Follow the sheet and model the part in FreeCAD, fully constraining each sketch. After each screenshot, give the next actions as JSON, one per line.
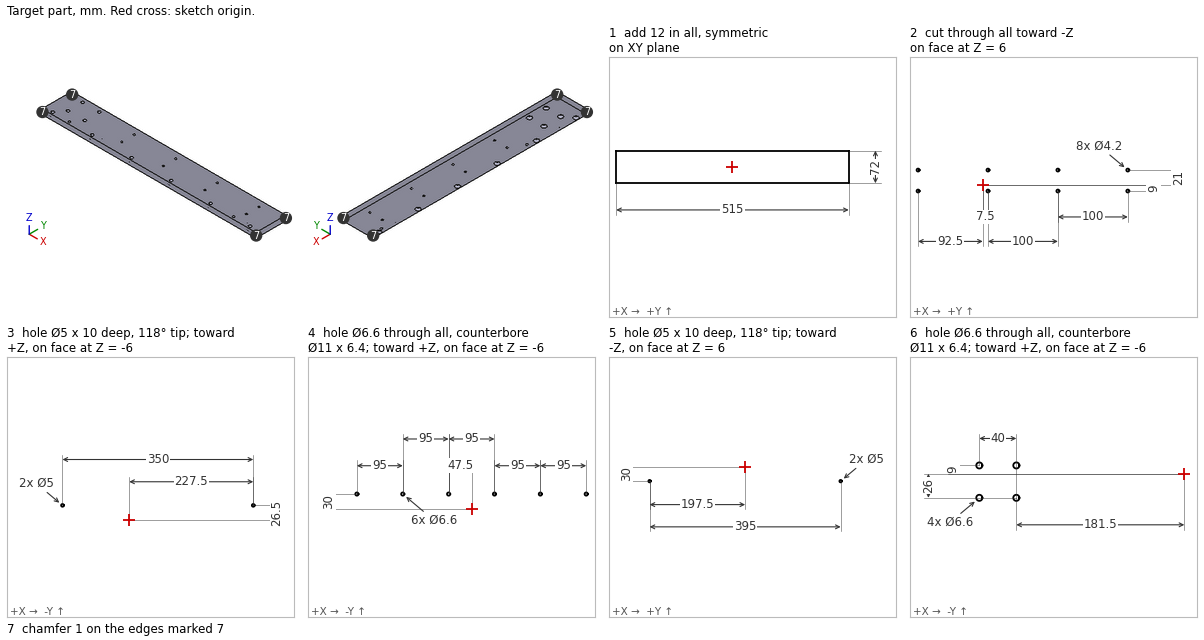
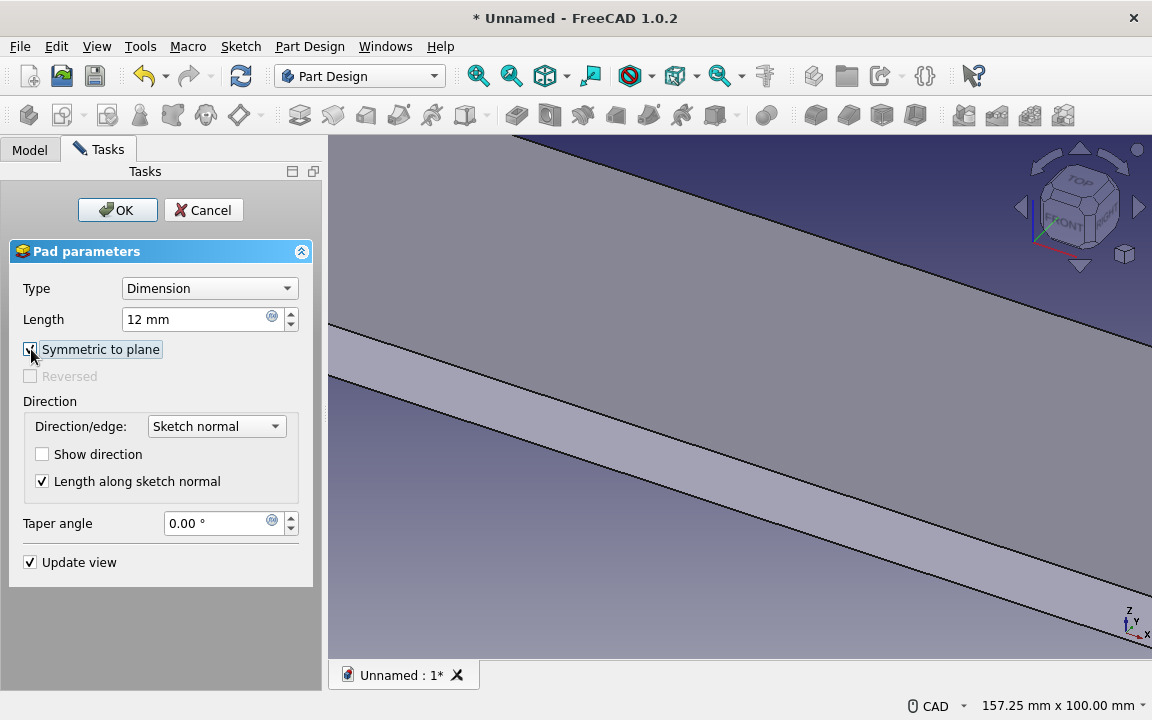
{"action": "left_click", "coordinate": [118, 210]}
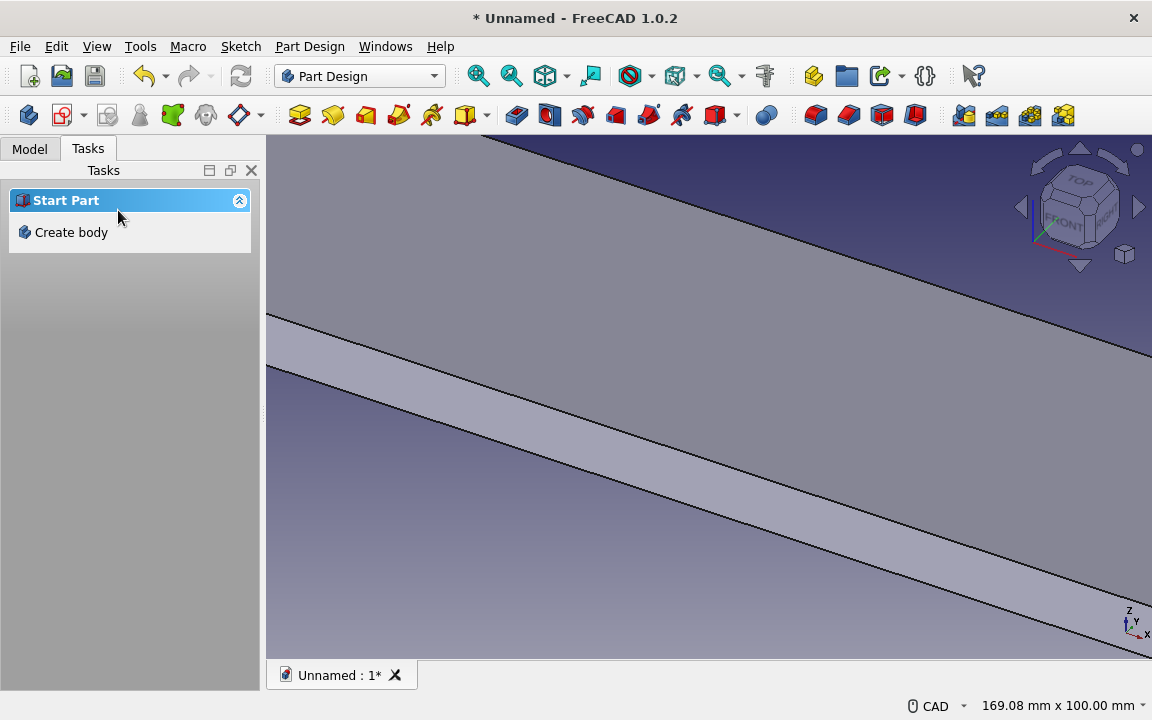
{"action": "left_click", "coordinate": [479, 76]}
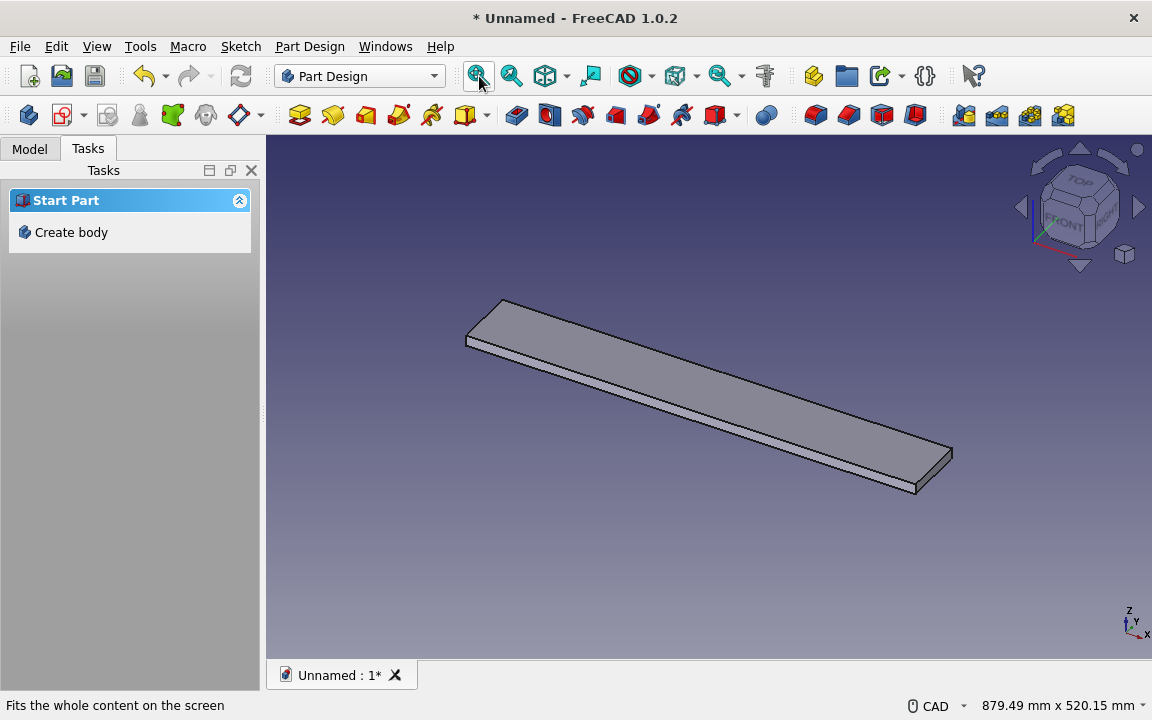
{"action": "left_click", "coordinate": [902, 455]}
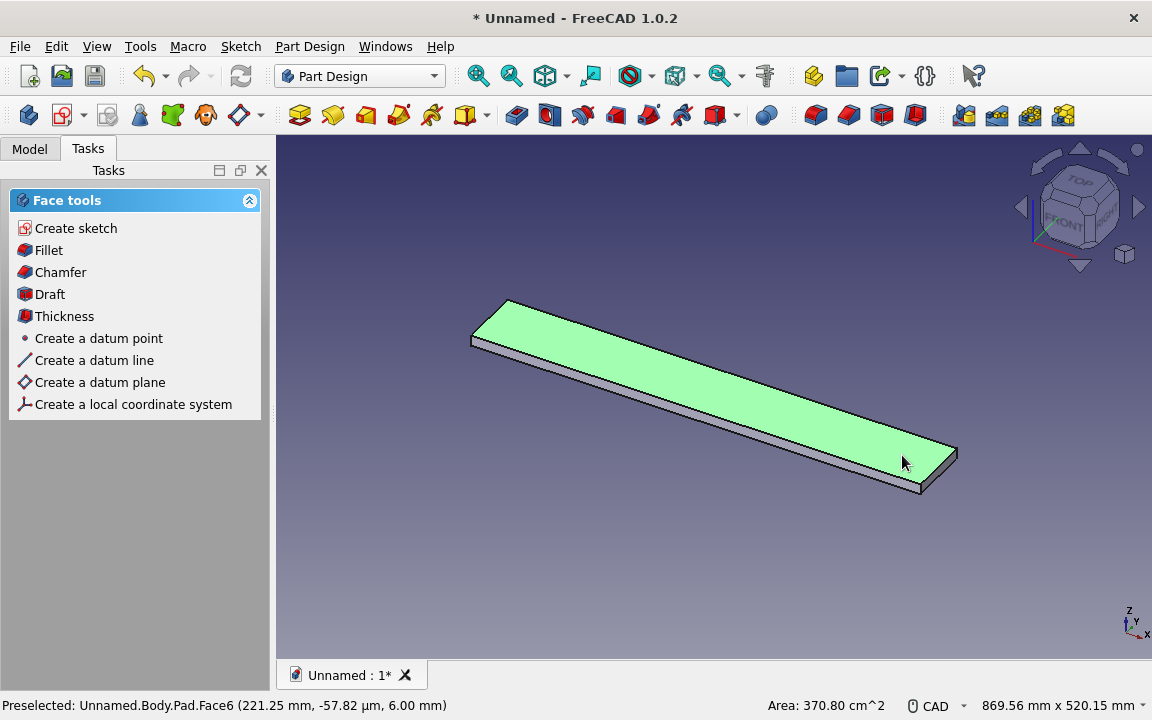
{"action": "left_click", "coordinate": [62, 116]}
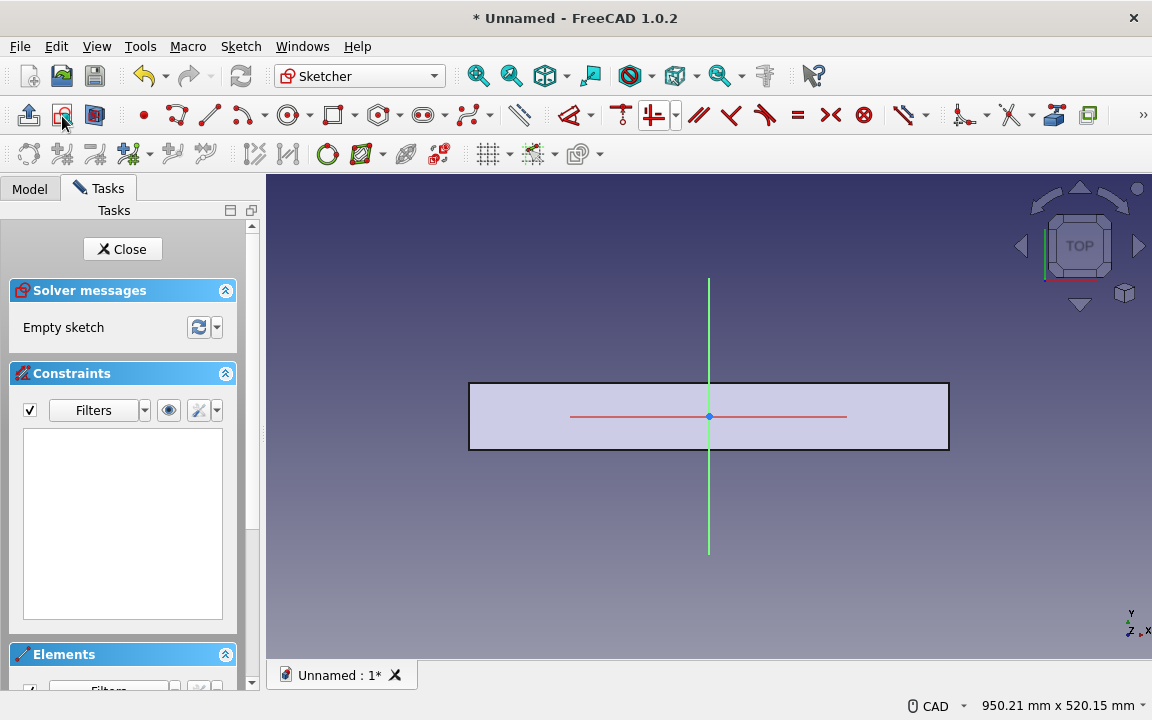
{"action": "scroll", "coordinate": [911, 404], "scroll_direction": "up", "scroll_amount": 3}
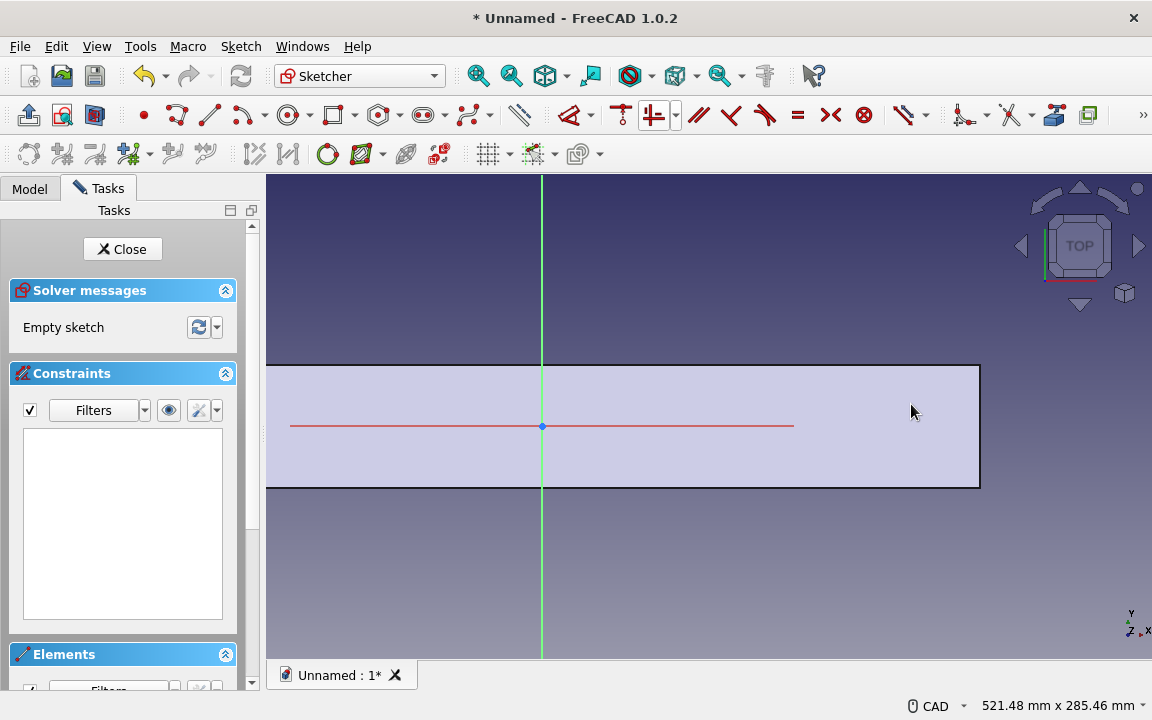
{"action": "left_click", "coordinate": [288, 116]}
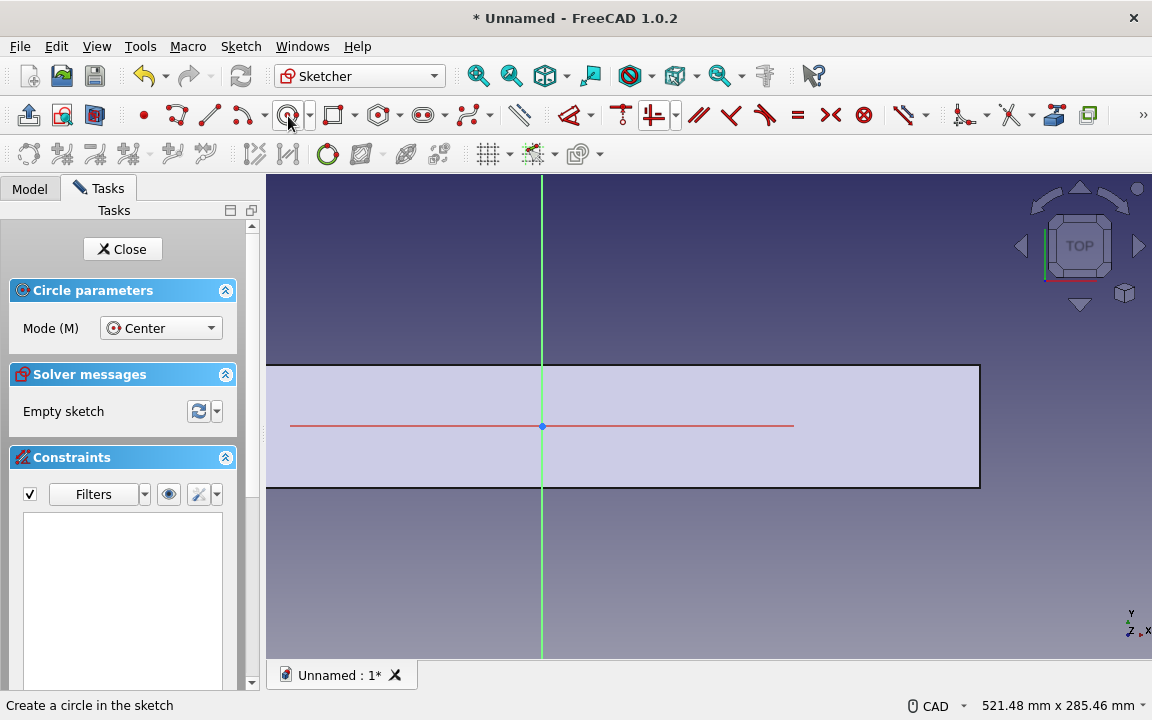
{"action": "scroll", "coordinate": [895, 442], "scroll_direction": "up", "scroll_amount": 10}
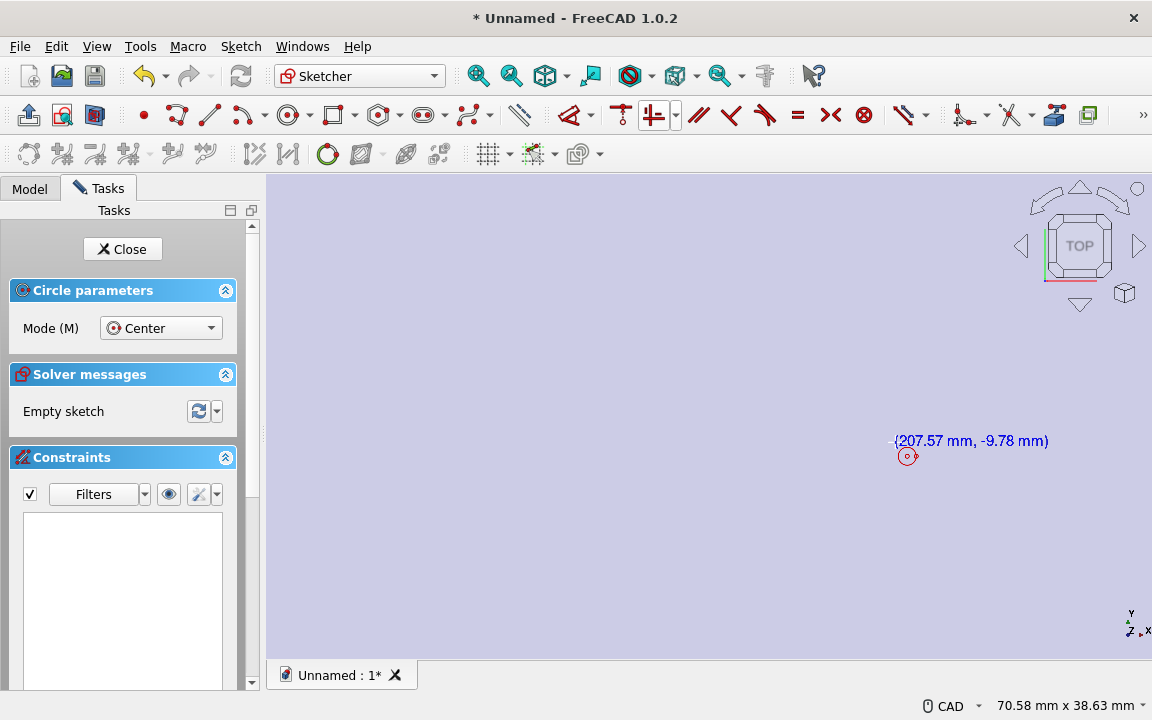
{"action": "scroll", "coordinate": [896, 443], "scroll_direction": "down", "scroll_amount": 10}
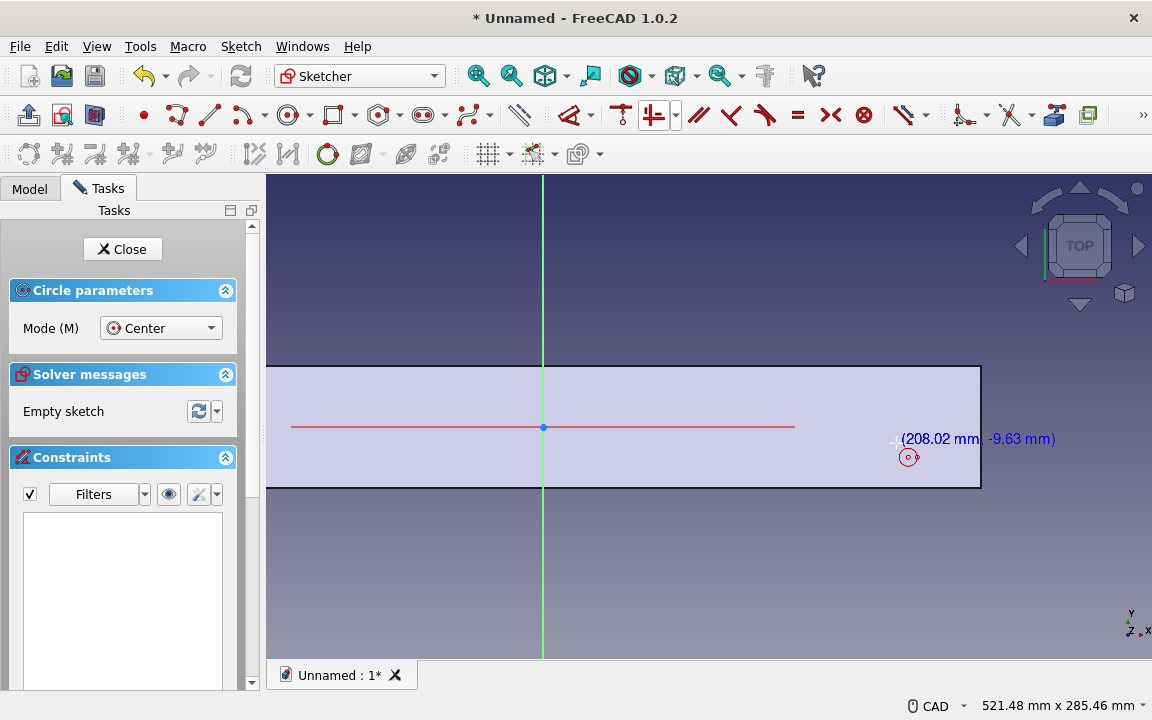
{"action": "left_click", "coordinate": [896, 443]}
{"action": "mouse_move", "coordinate": [898, 445]}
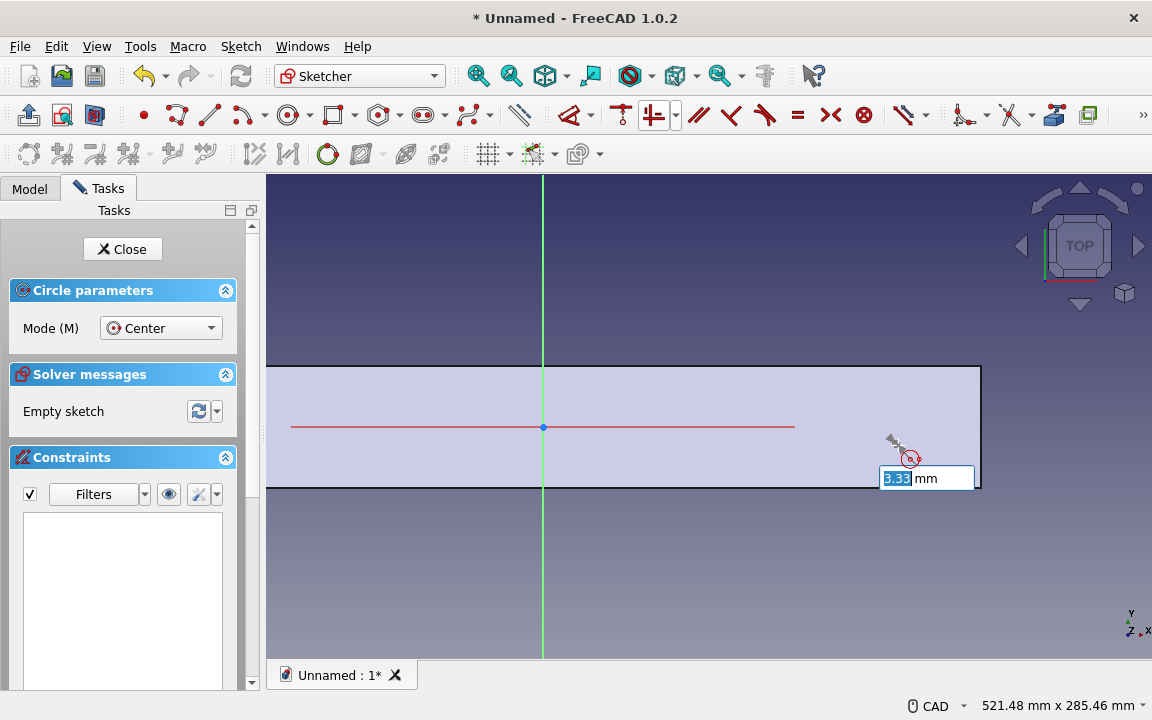
{"action": "type", "text": "4.2"}
{"action": "key", "text": "Return"}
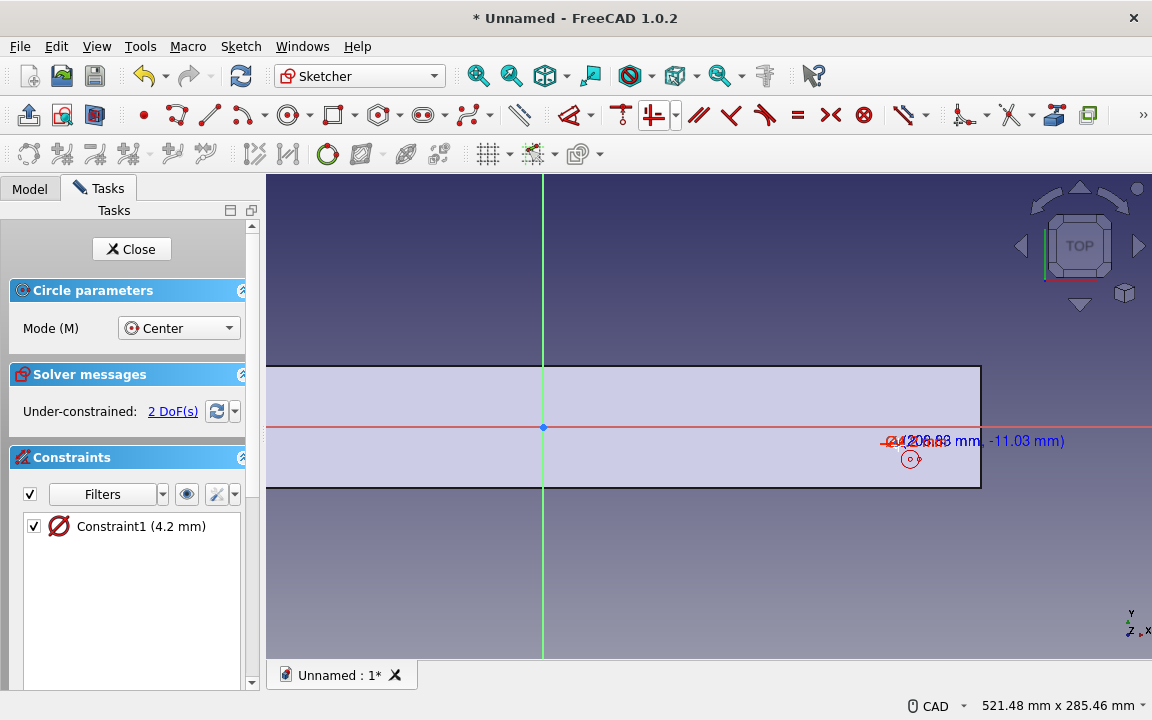
{"action": "scroll", "coordinate": [896, 392], "scroll_direction": "up", "scroll_amount": 10}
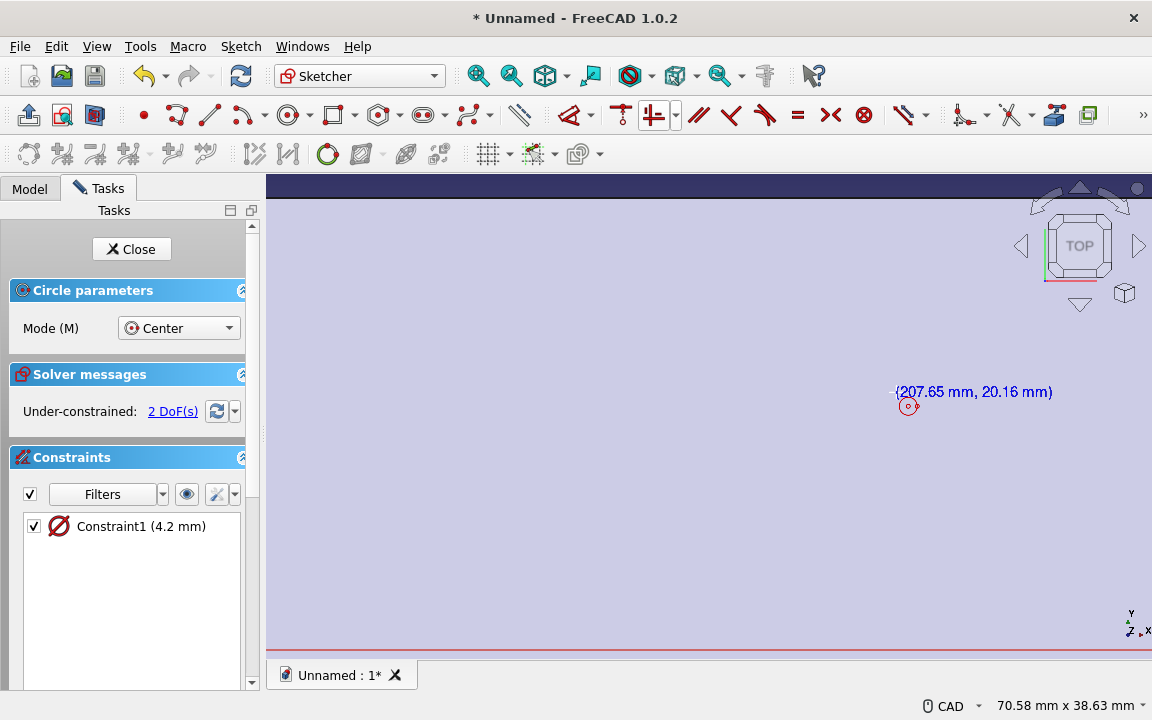
{"action": "scroll", "coordinate": [896, 392], "scroll_direction": "down", "scroll_amount": 10}